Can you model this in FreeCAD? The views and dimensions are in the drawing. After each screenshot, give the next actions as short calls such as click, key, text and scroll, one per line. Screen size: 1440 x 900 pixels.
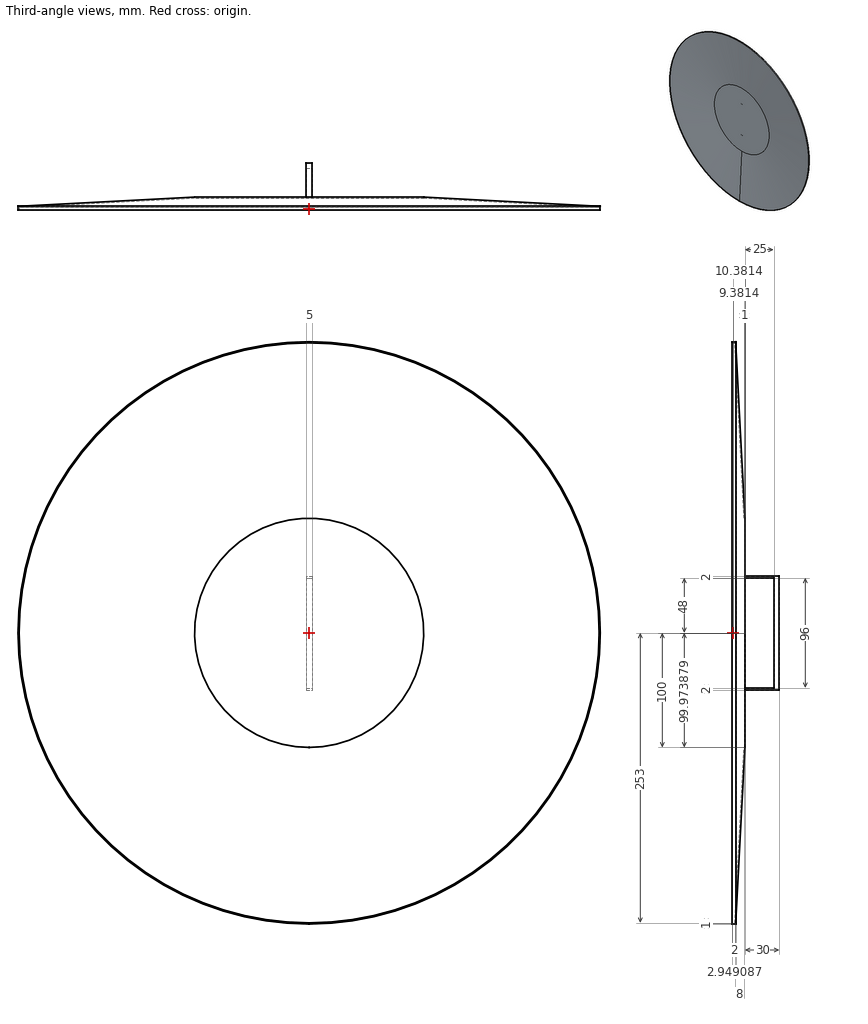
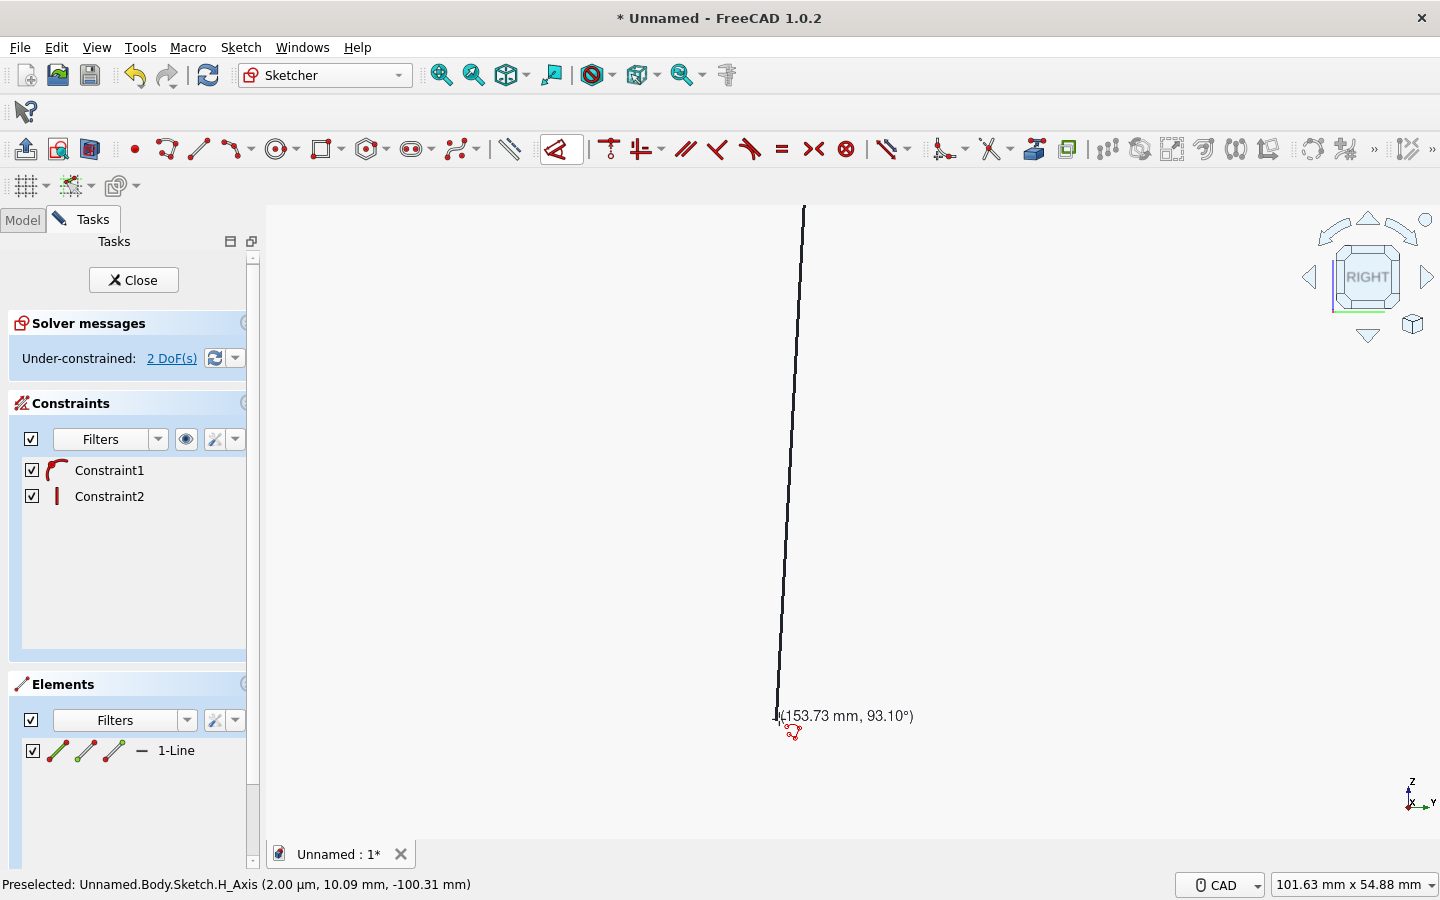
click(779, 712)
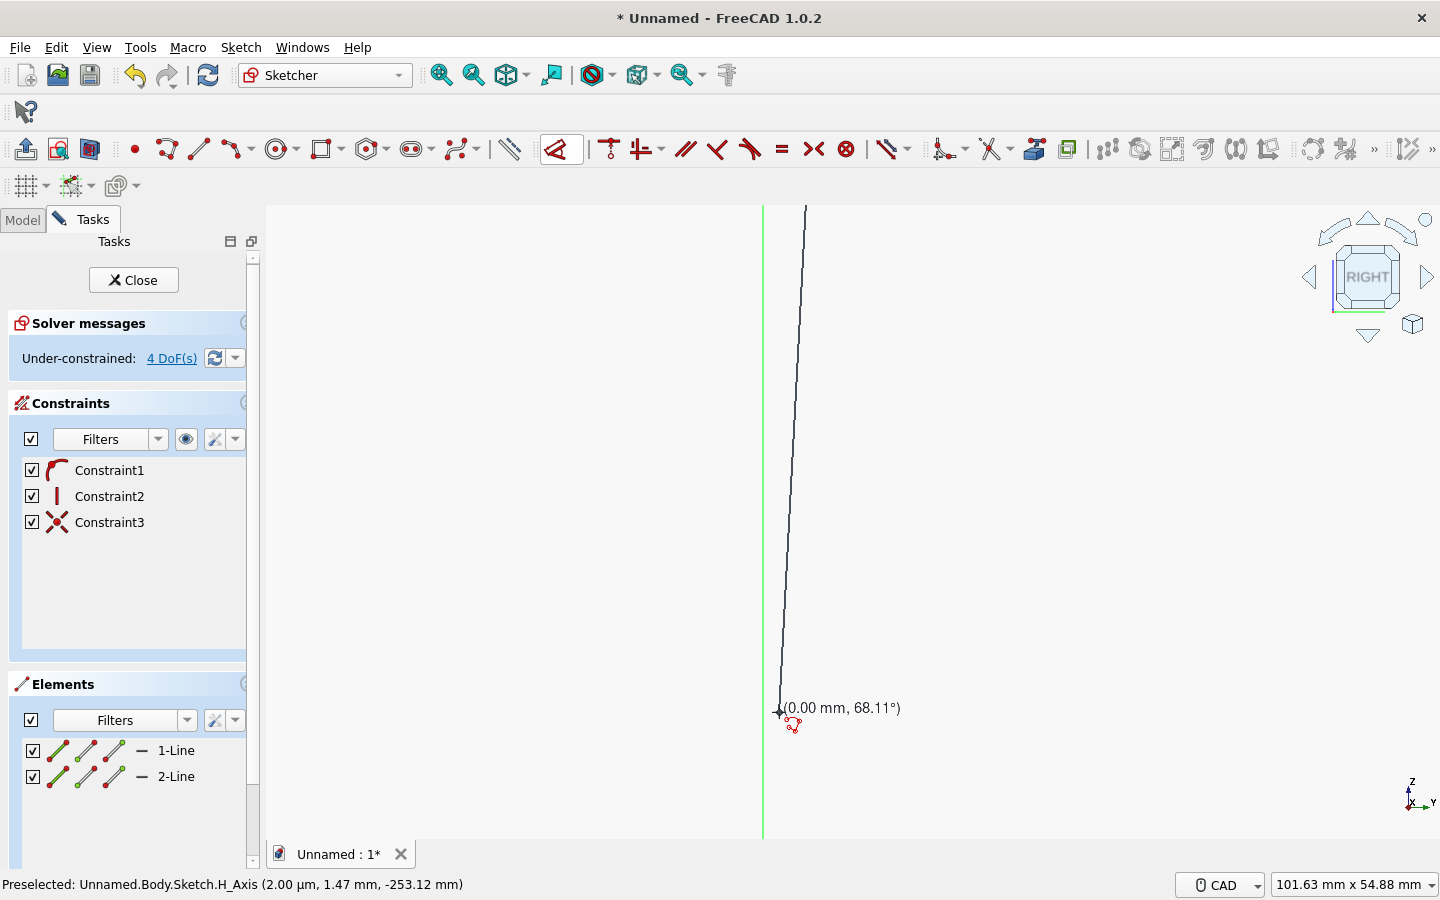
scroll(756, 712, up, 4)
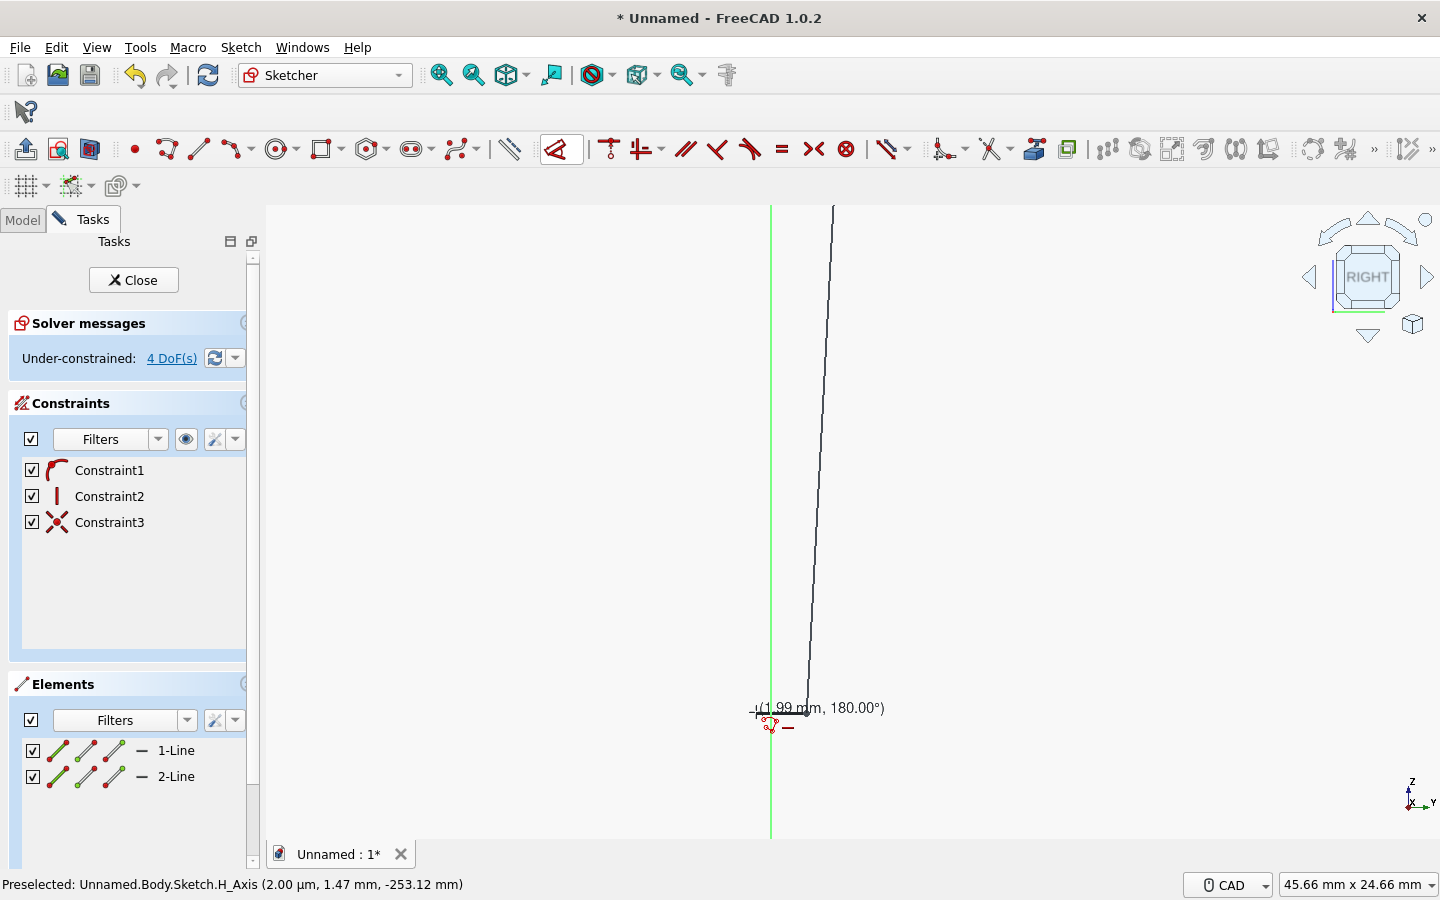
click(755, 711)
click(755, 736)
click(831, 736)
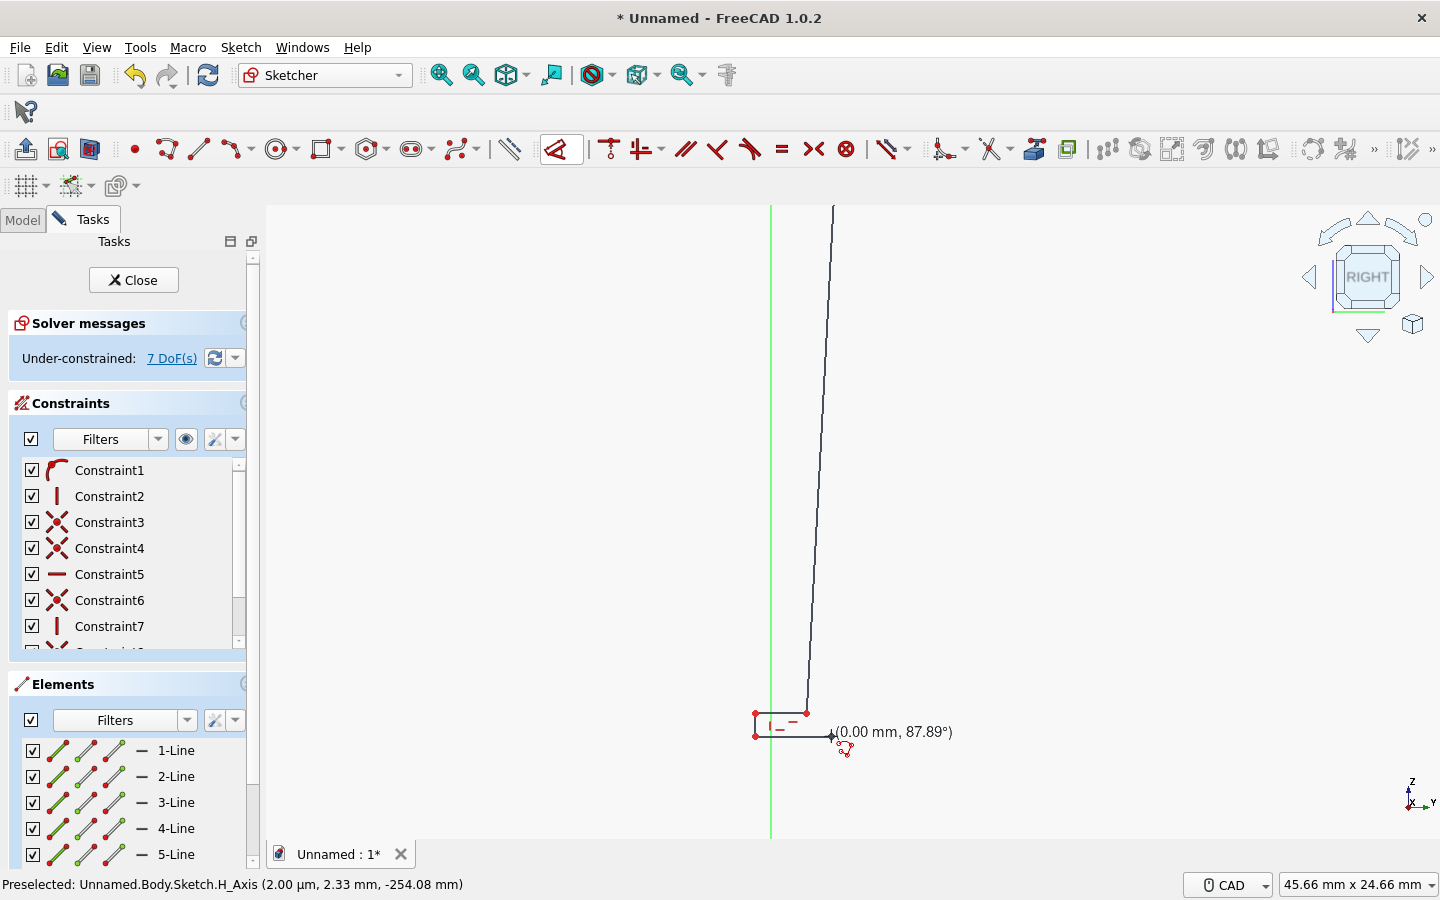
scroll(777, 720, down, 14)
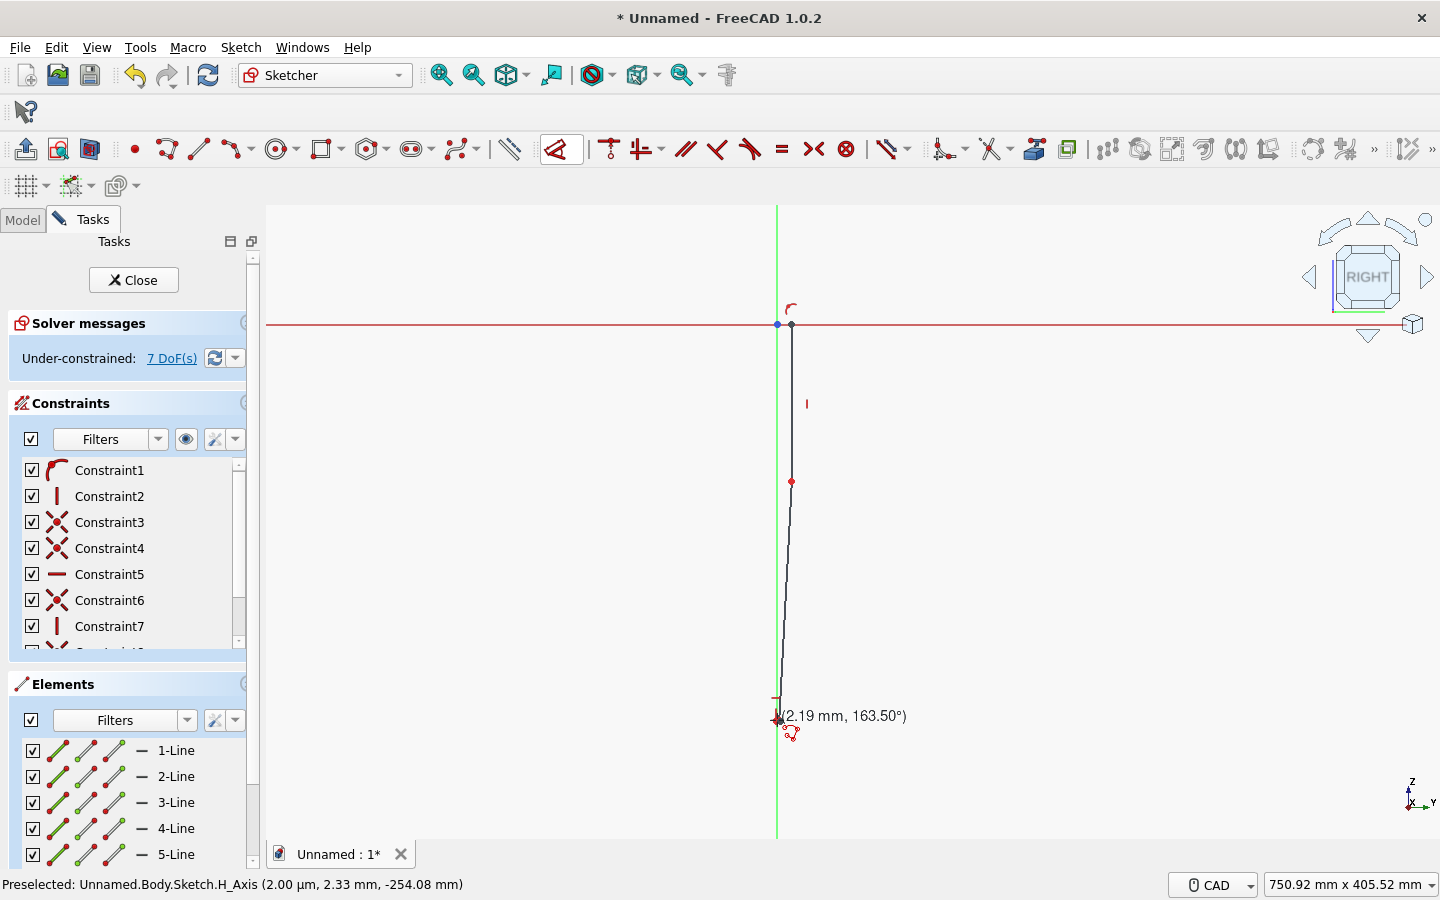
scroll(793, 481, up, 12)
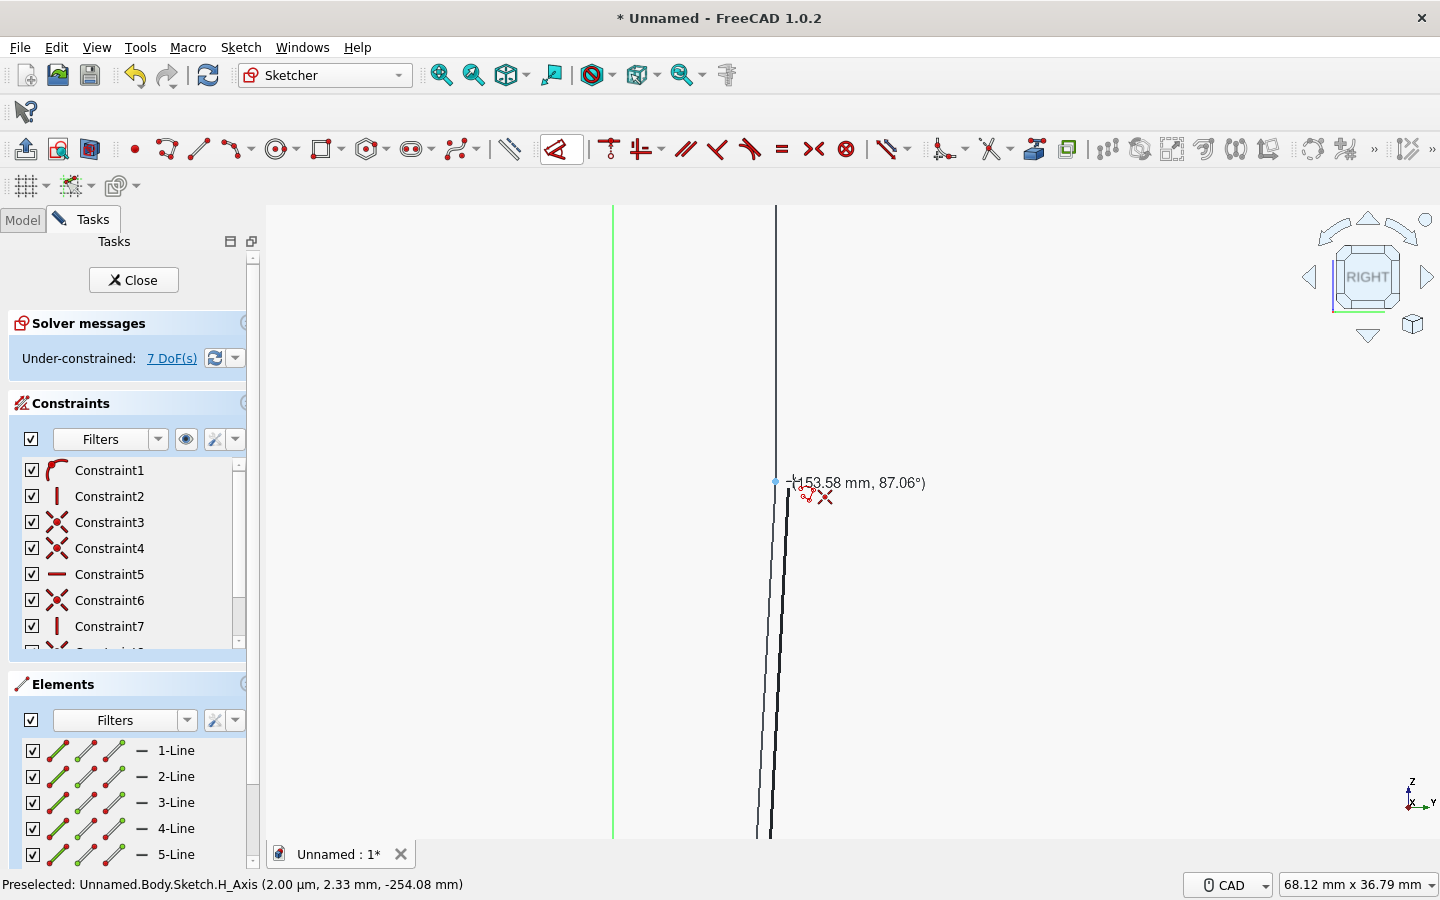
click(792, 476)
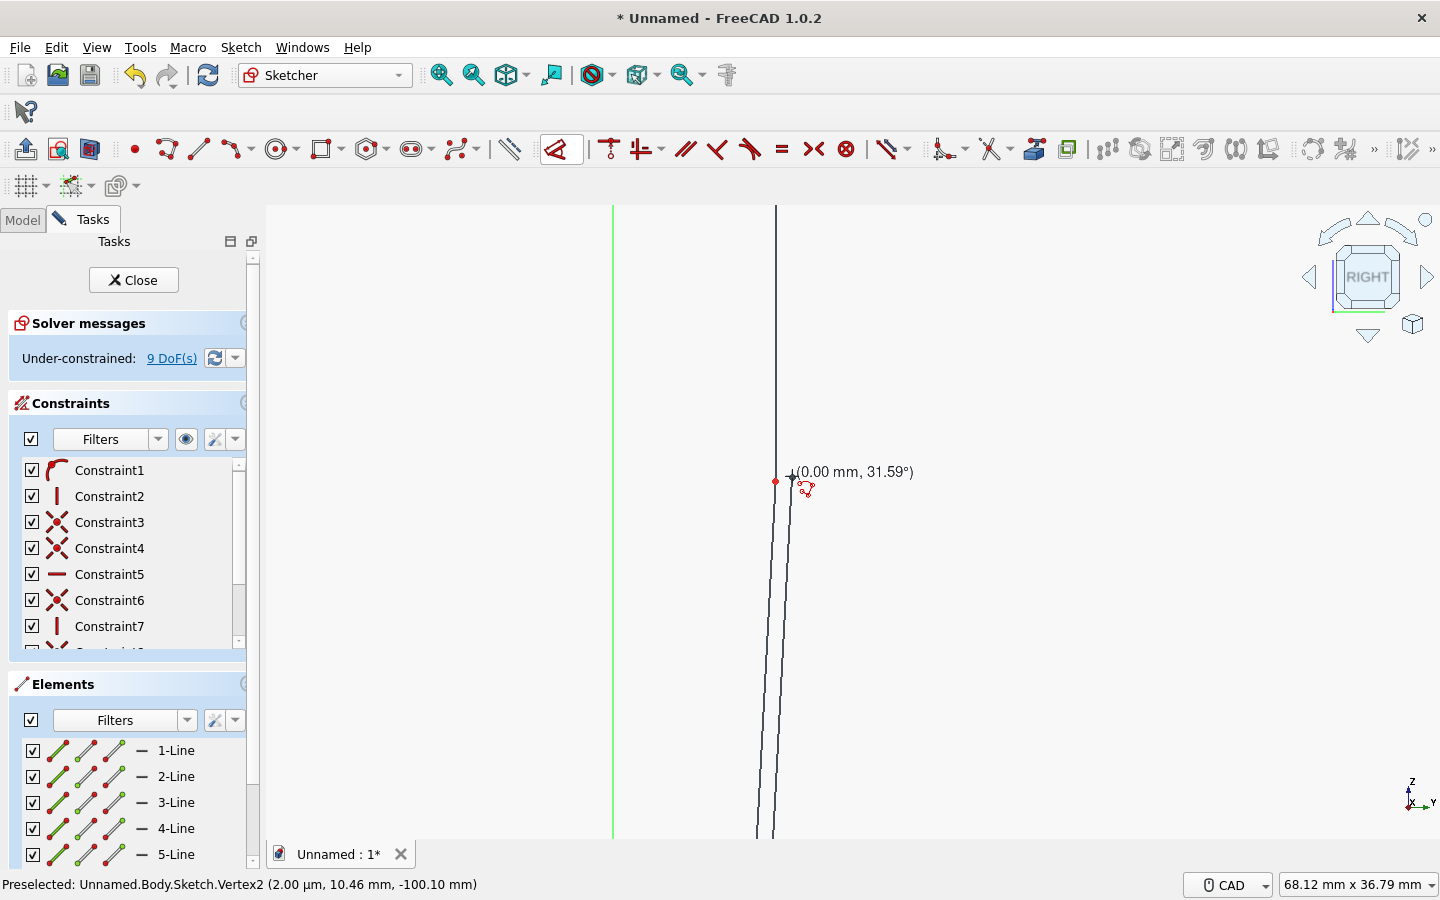
scroll(793, 480, down, 12)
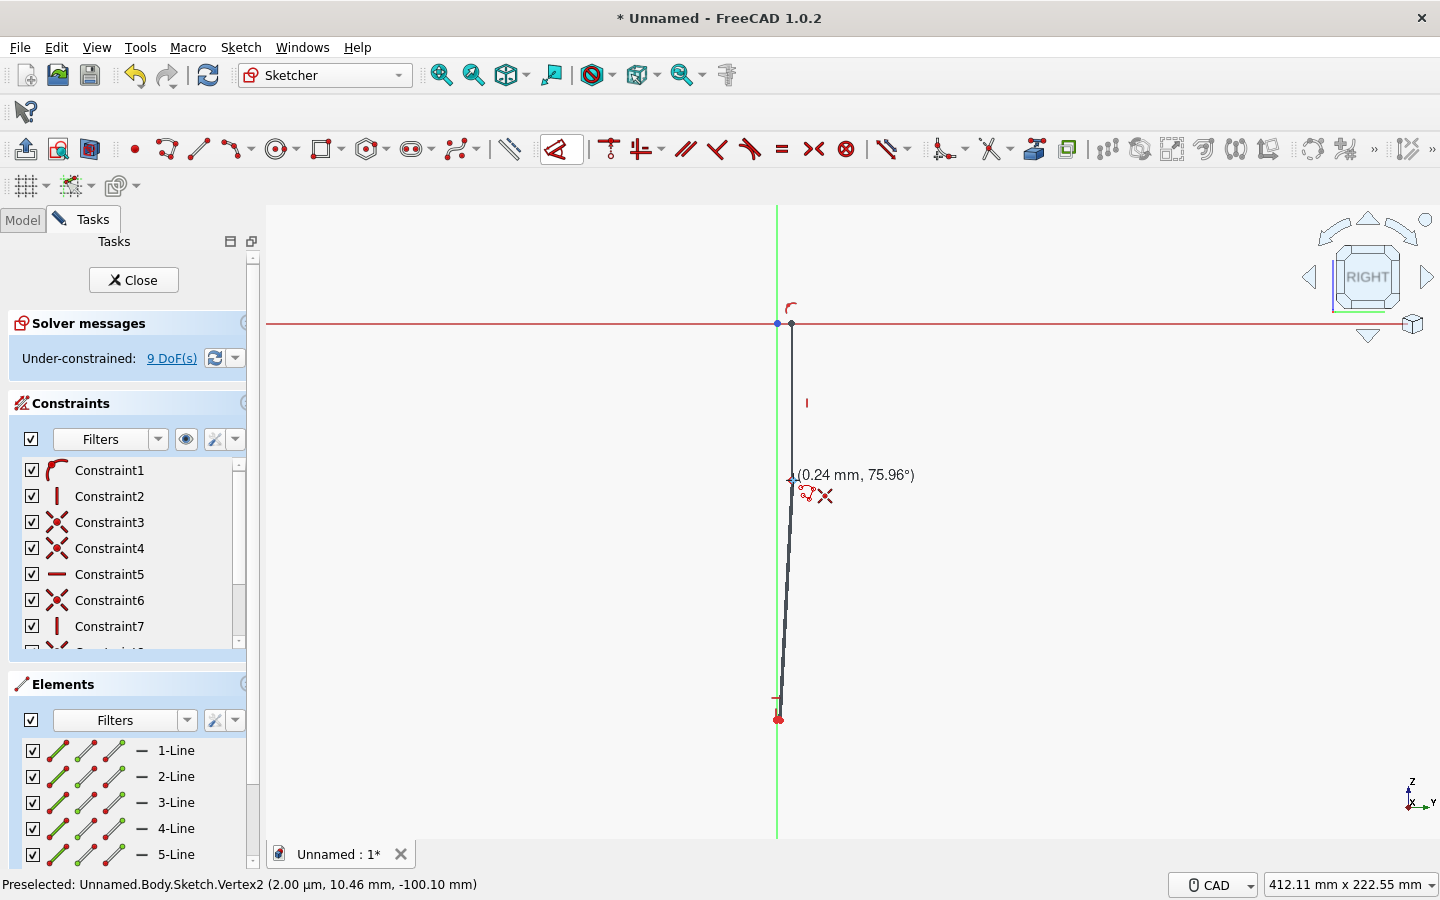
scroll(793, 324, up, 12)